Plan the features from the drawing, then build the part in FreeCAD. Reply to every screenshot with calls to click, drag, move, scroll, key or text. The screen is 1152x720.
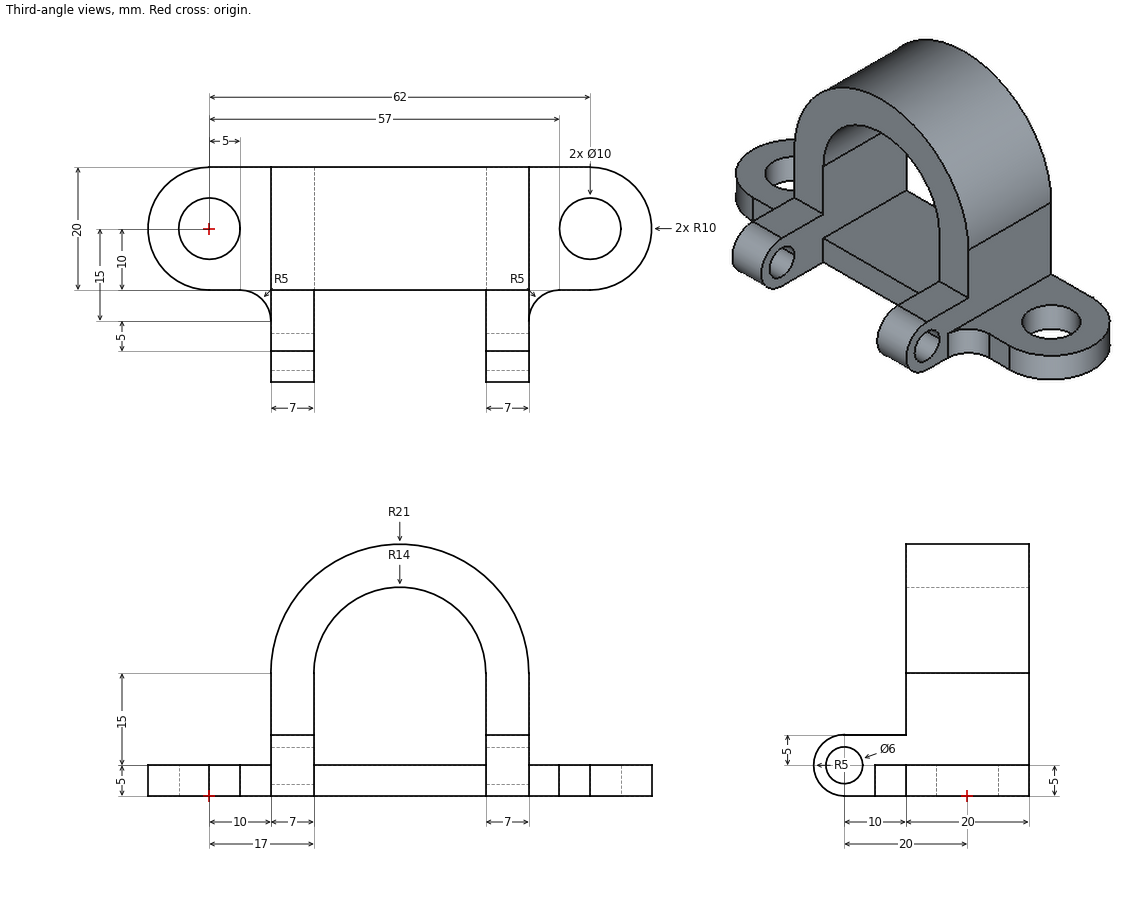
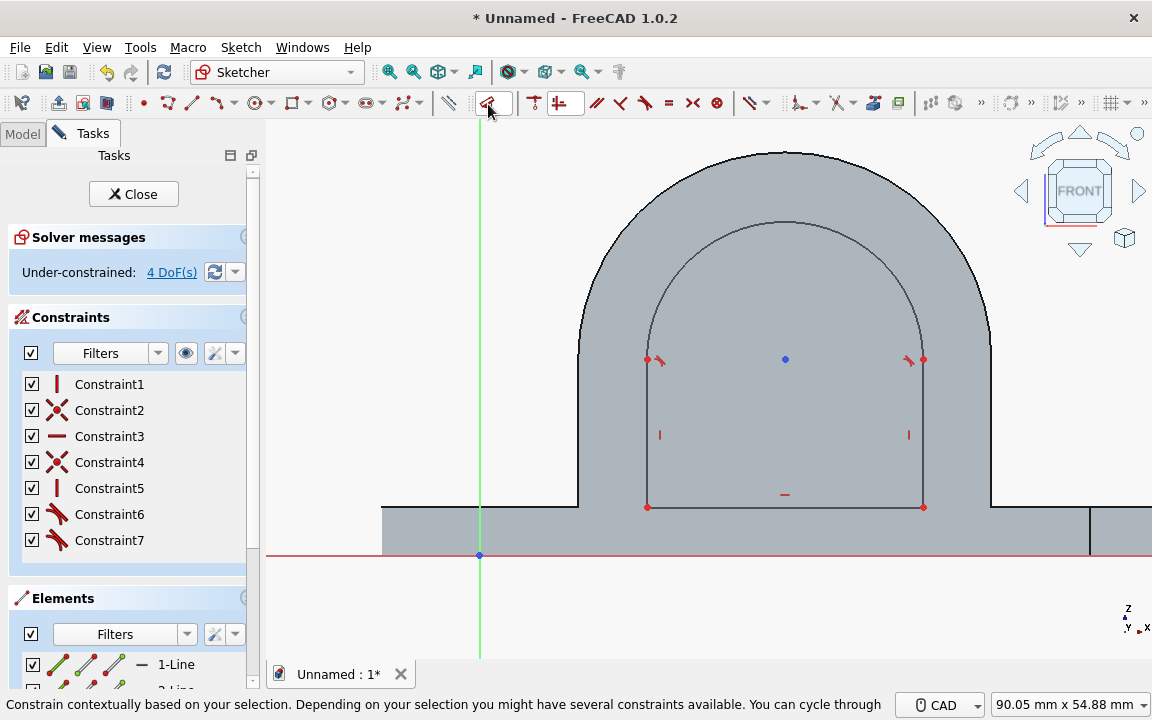
click(866, 248)
click(885, 222)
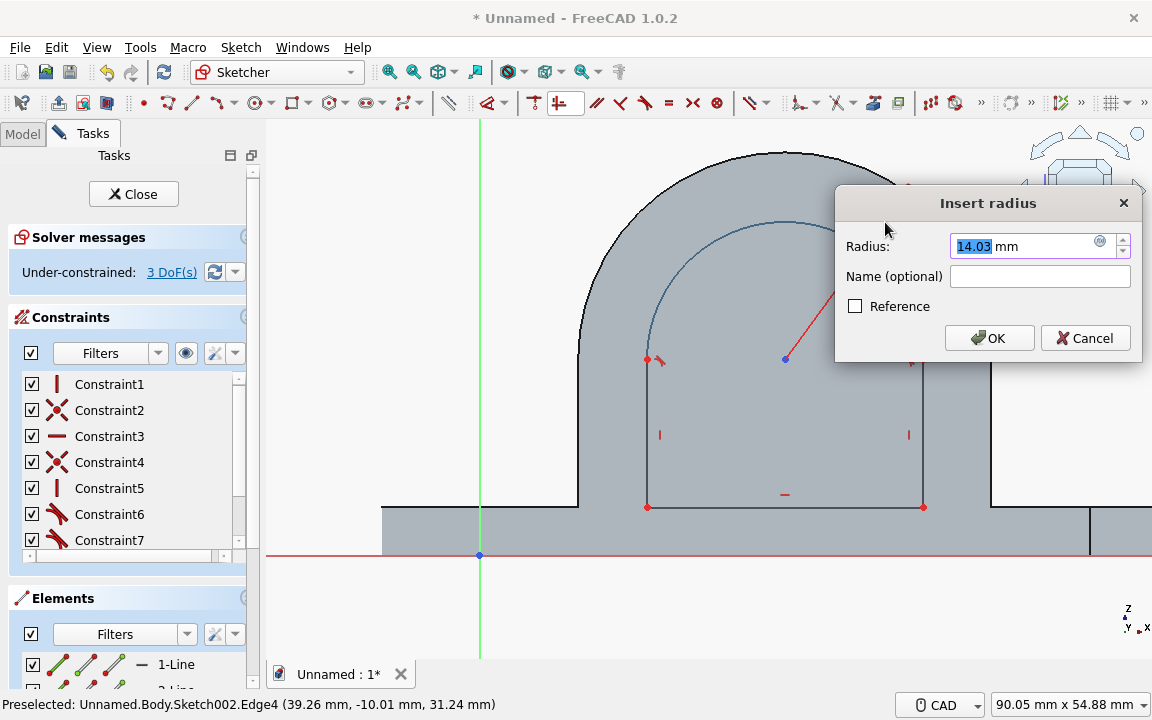
text(14)
key(Return)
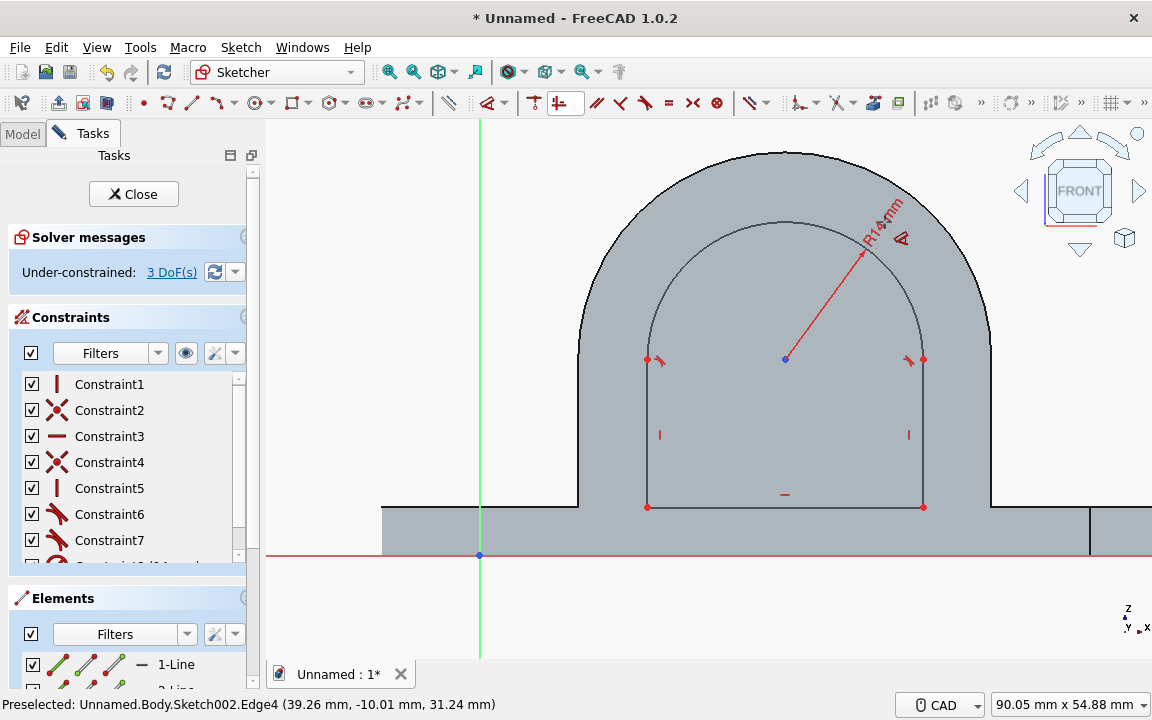
click(647, 404)
click(613, 434)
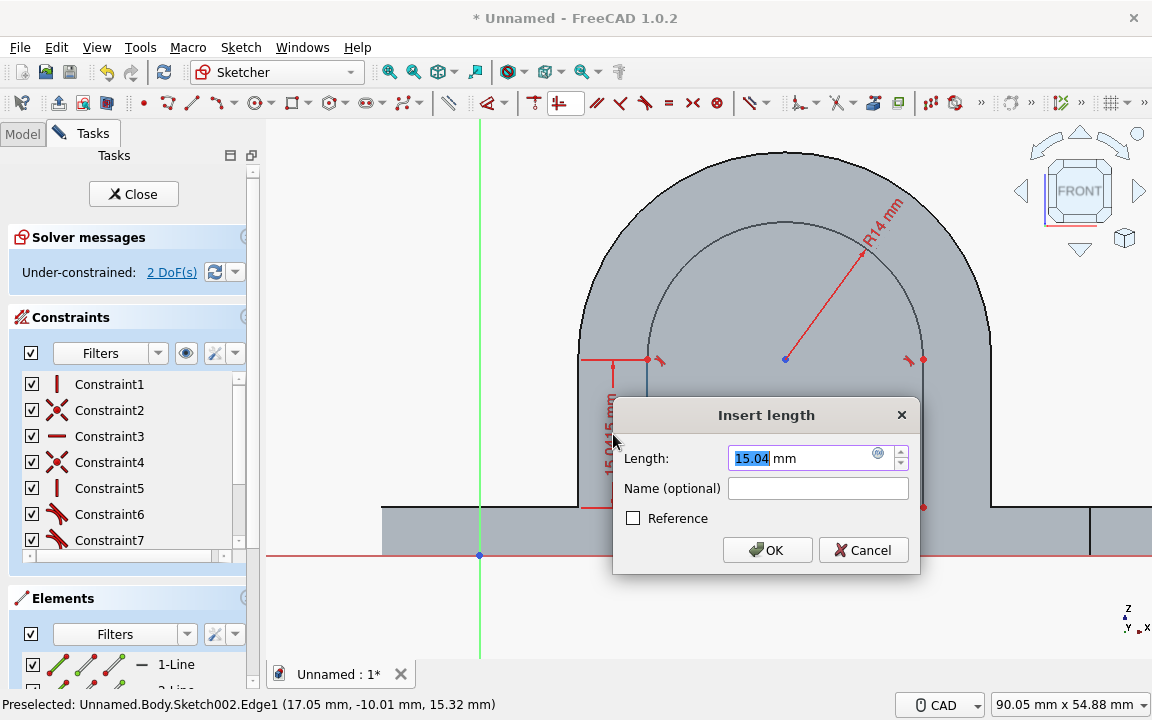
text(15)
key(Return)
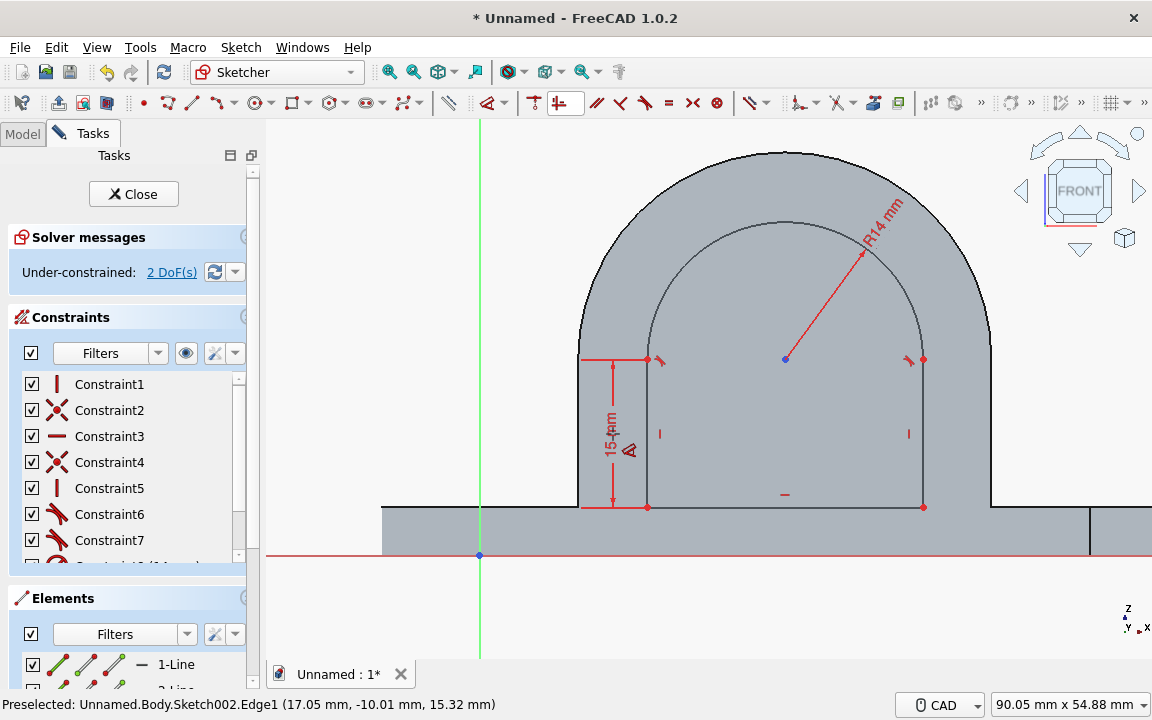
click(647, 508)
click(446, 532)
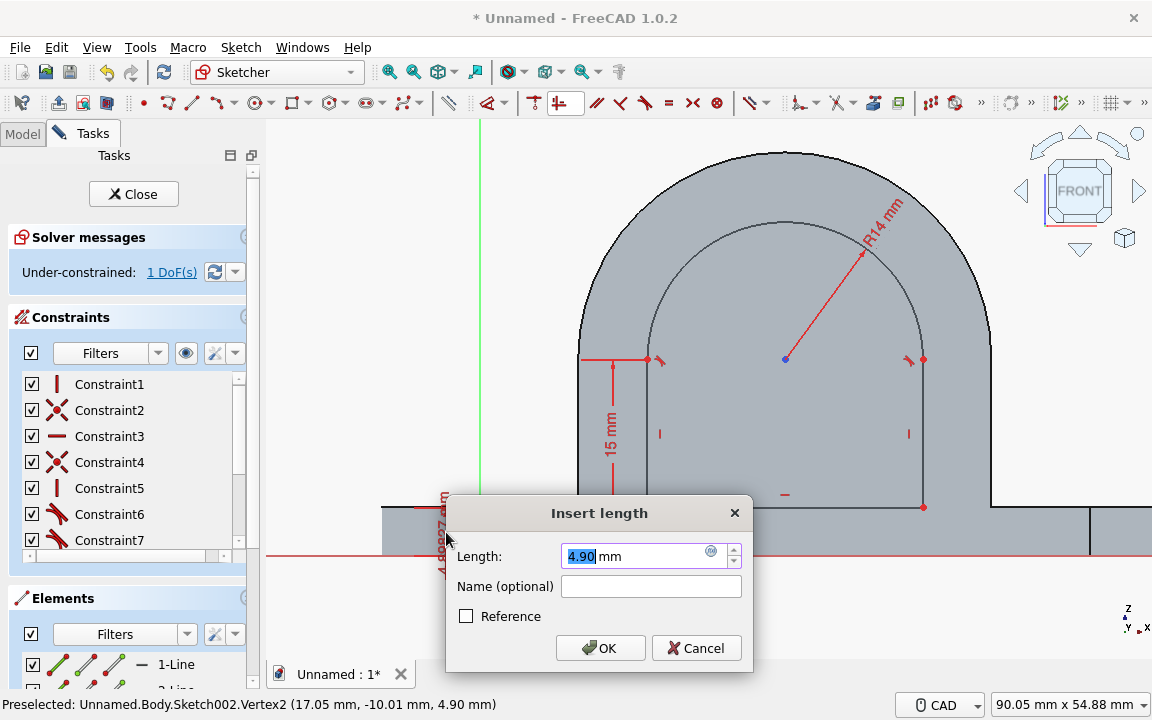
text(5)
key(Return)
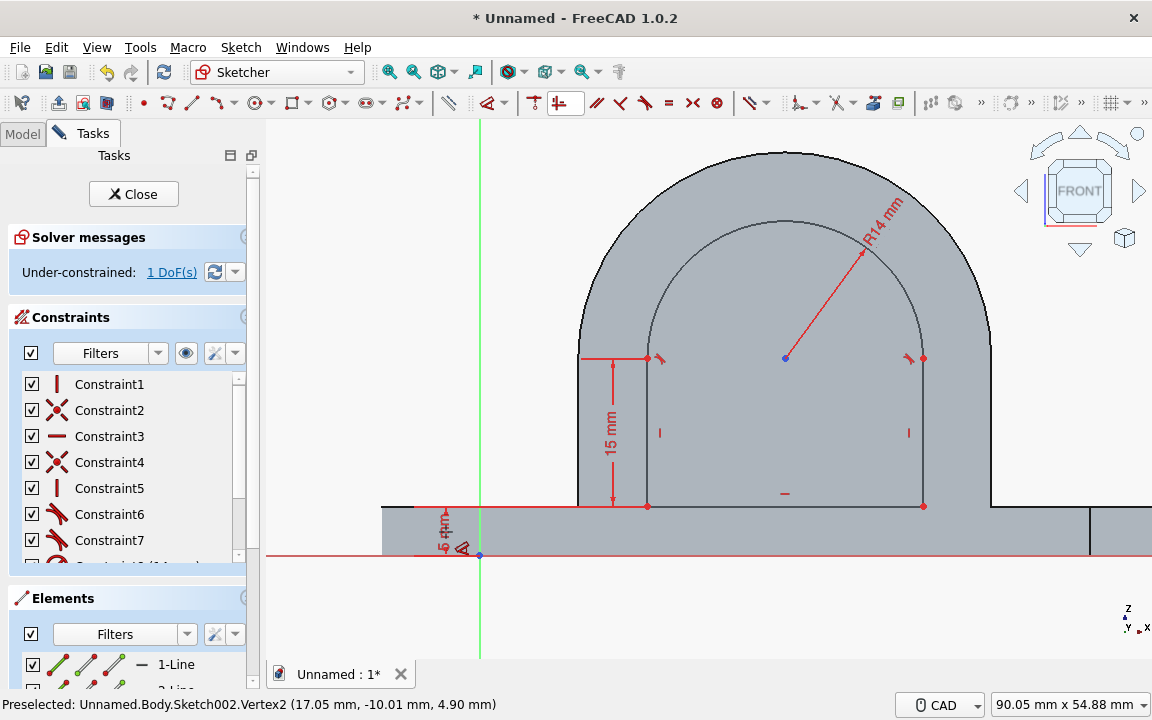
click(647, 359)
click(564, 590)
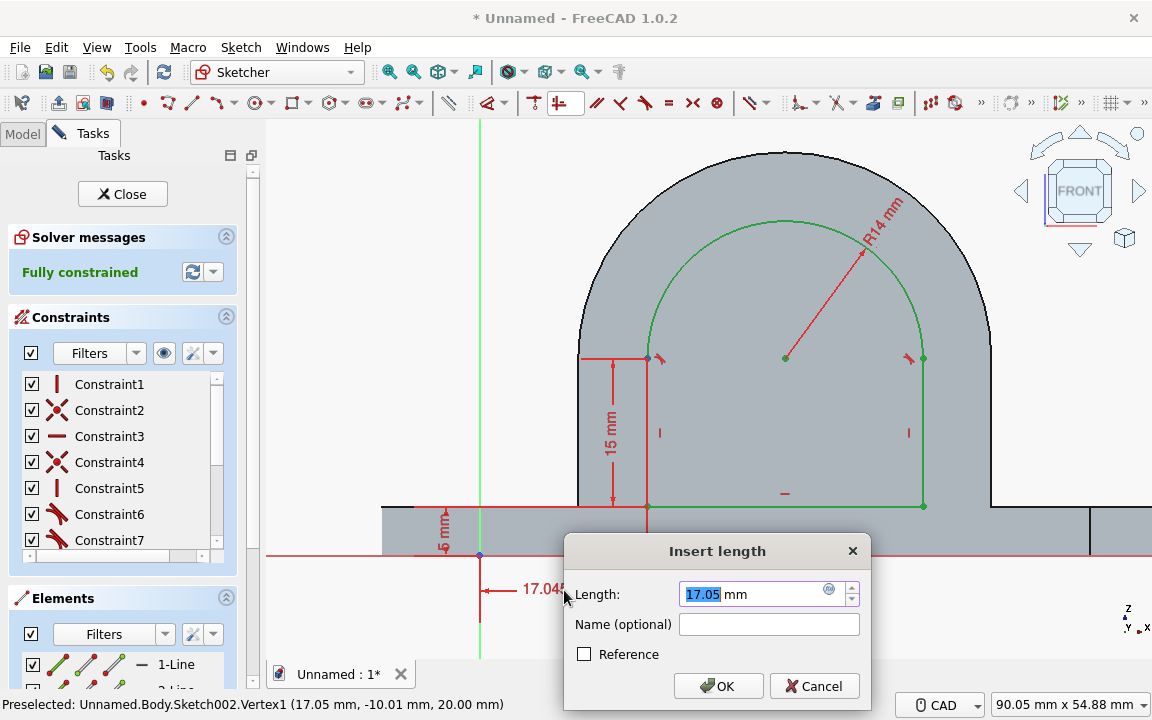
text(17)
key(Return)
key(Escape)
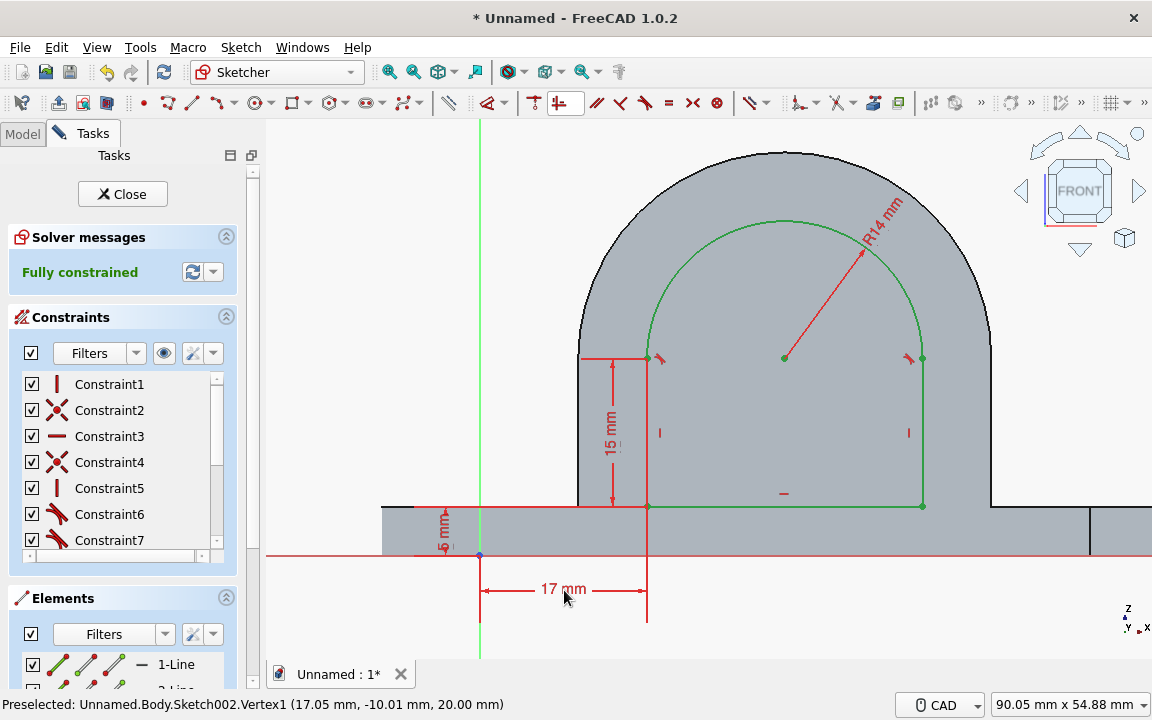
click(123, 194)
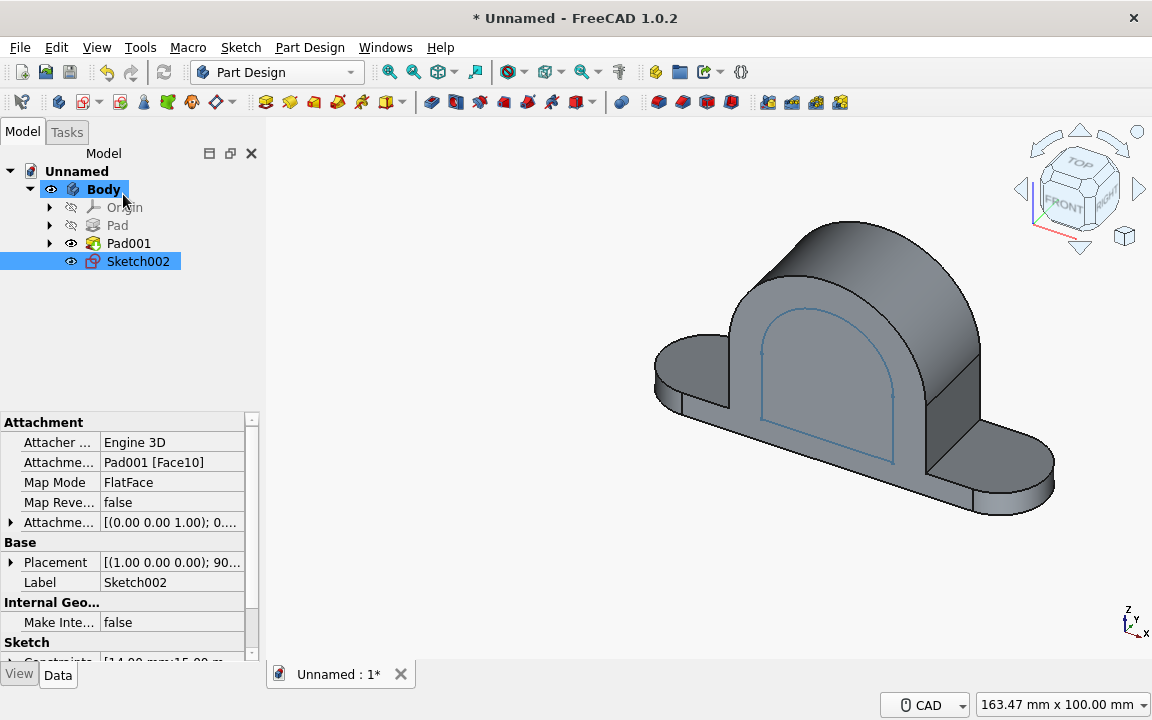
click(432, 102)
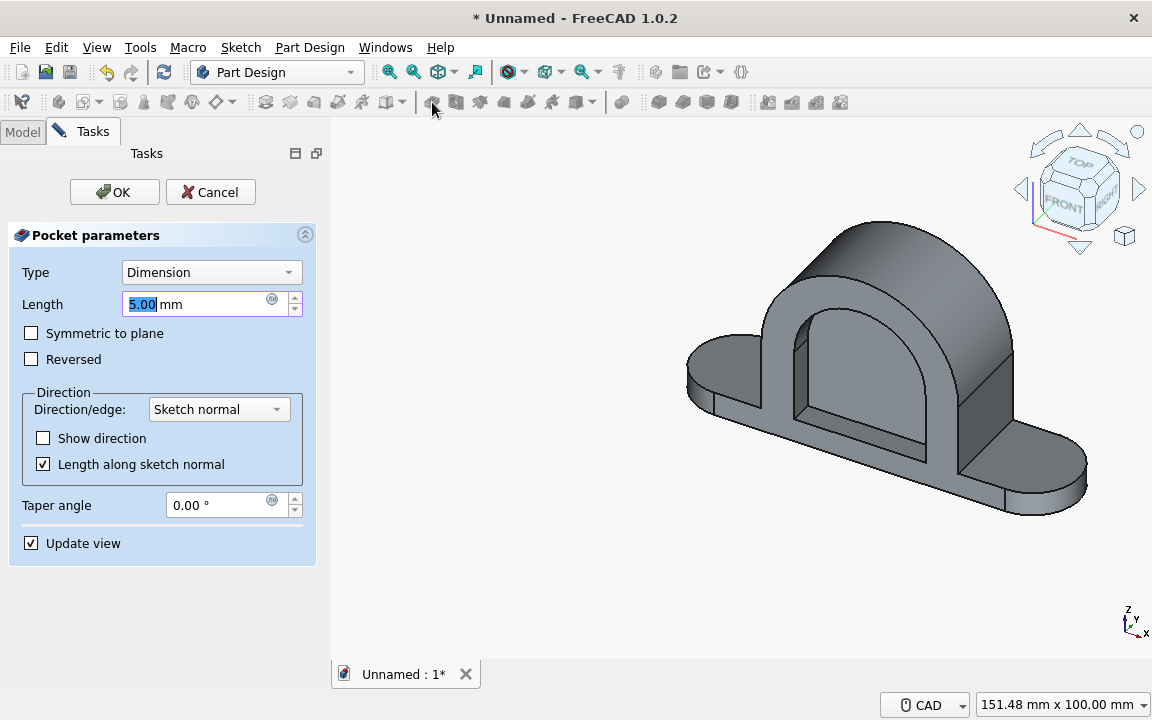
text(20)
key(Tab)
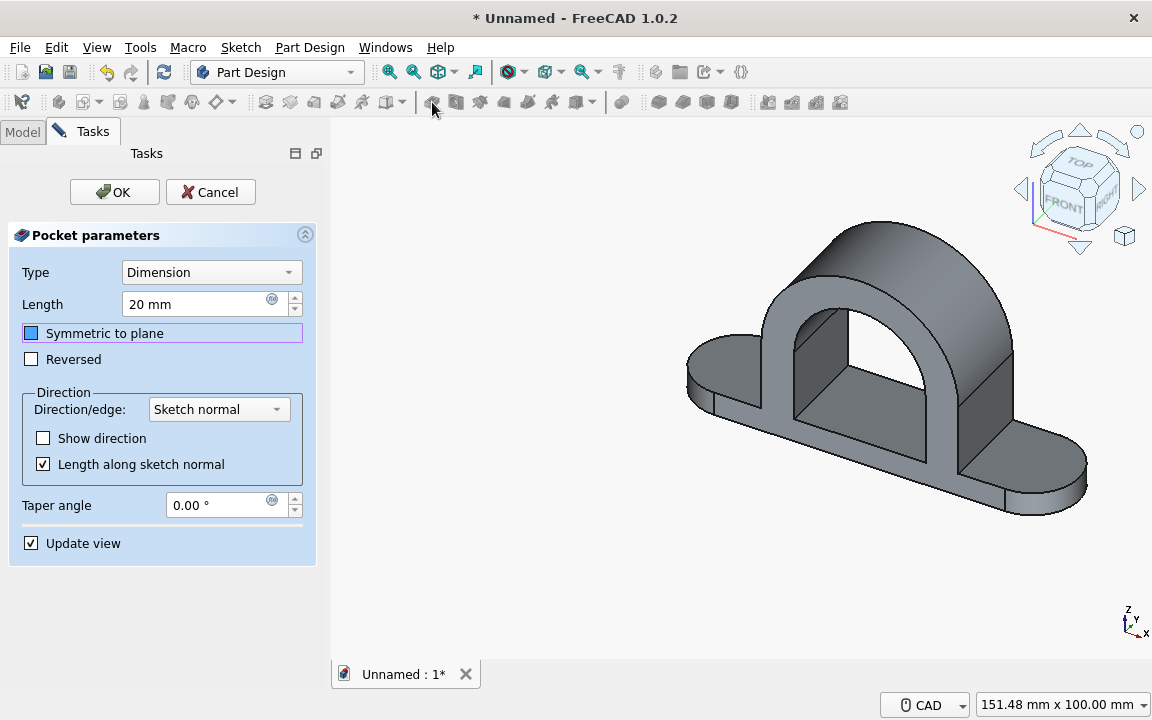
click(115, 192)